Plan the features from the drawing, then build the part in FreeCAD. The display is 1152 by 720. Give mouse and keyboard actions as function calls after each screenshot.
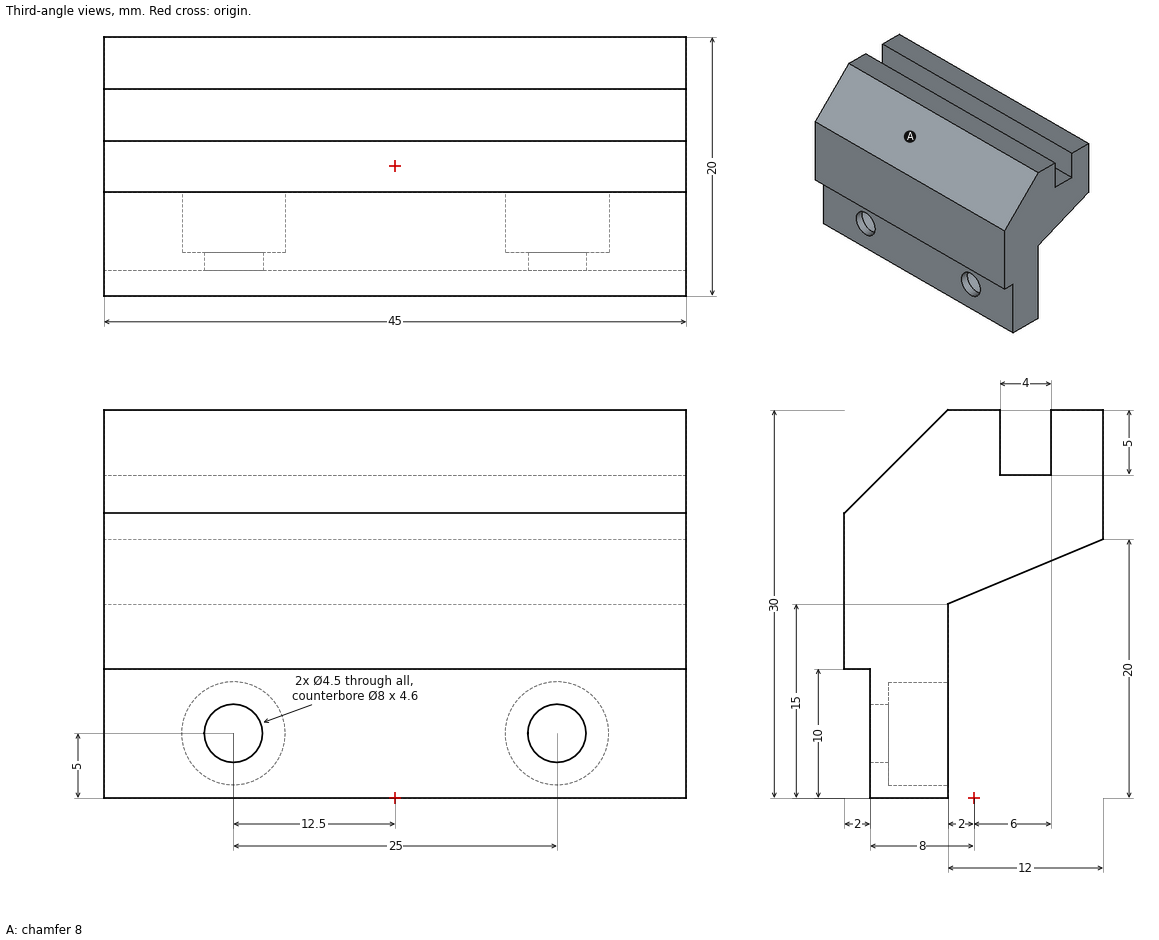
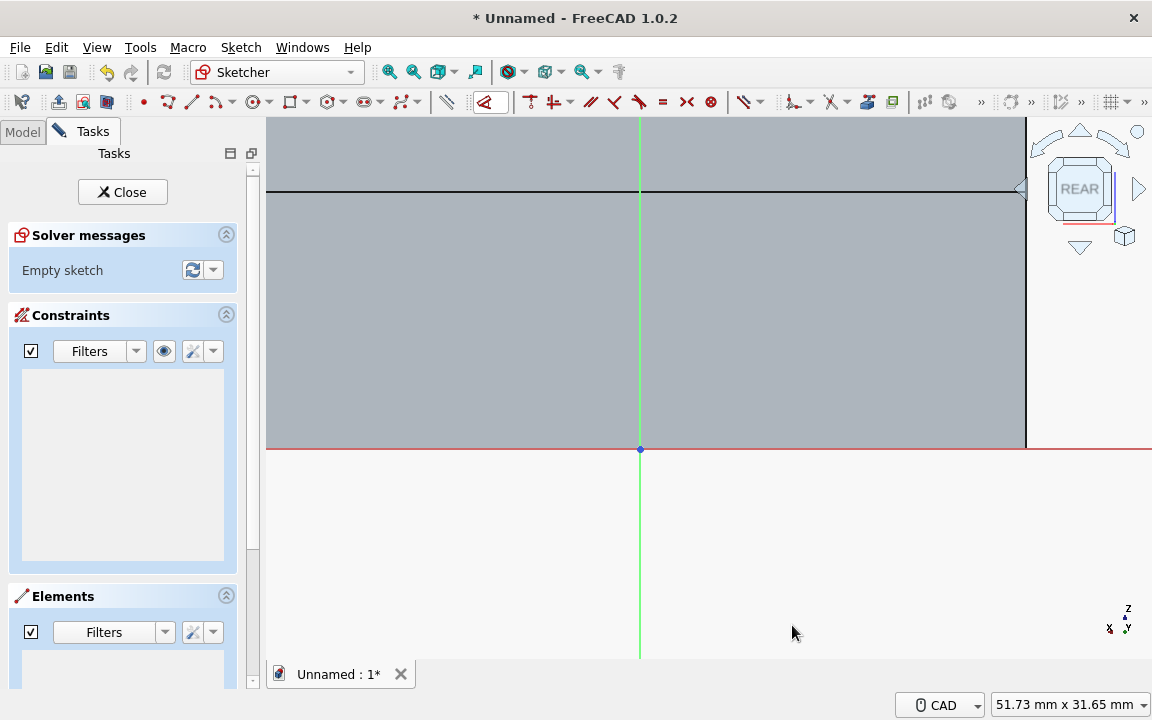
click(254, 102)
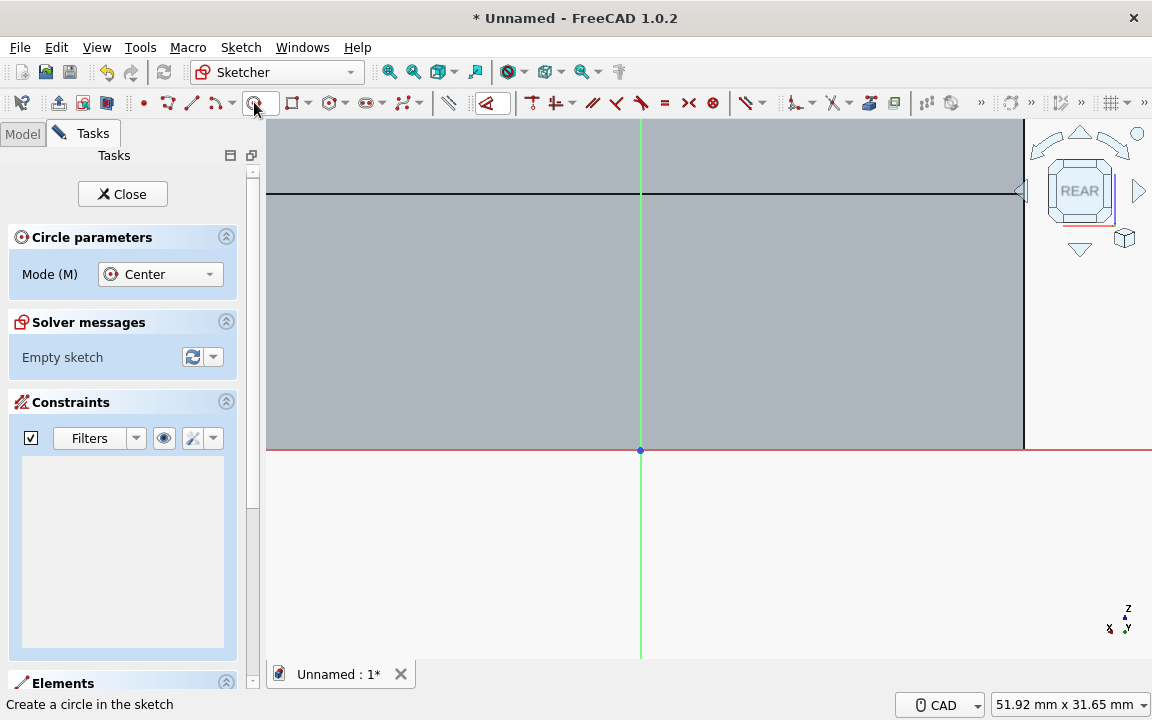
click(854, 365)
move(881, 338)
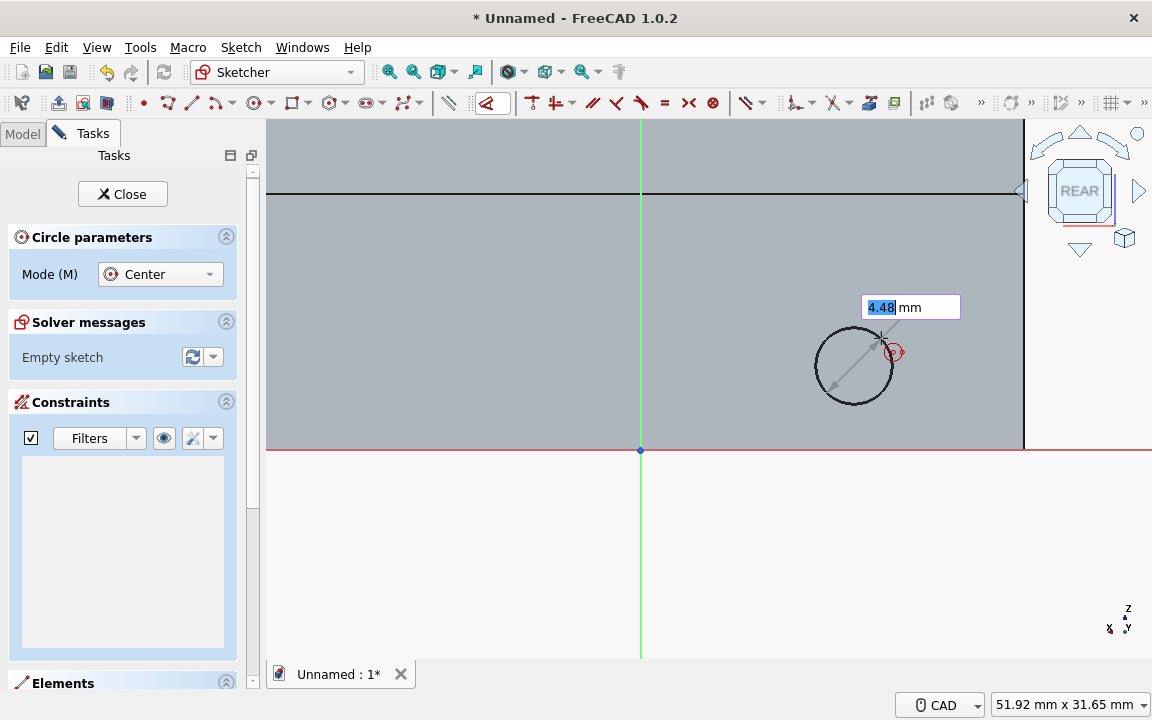
text(4.5)
key(Return)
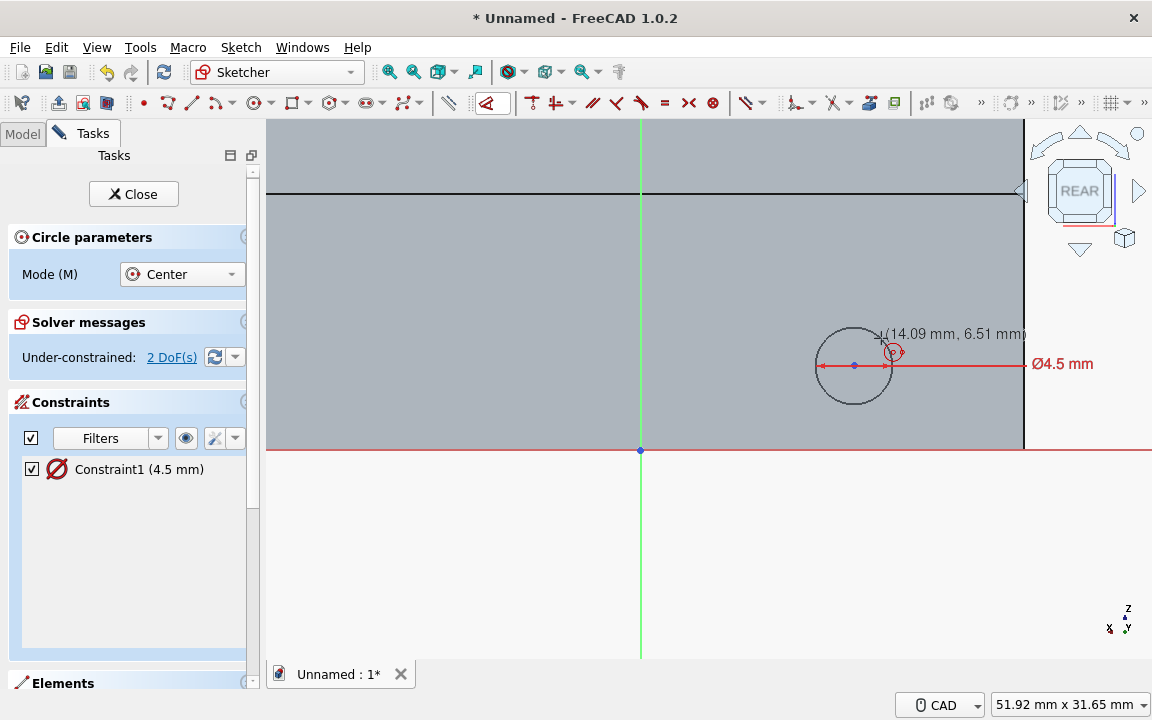
click(427, 365)
move(454, 338)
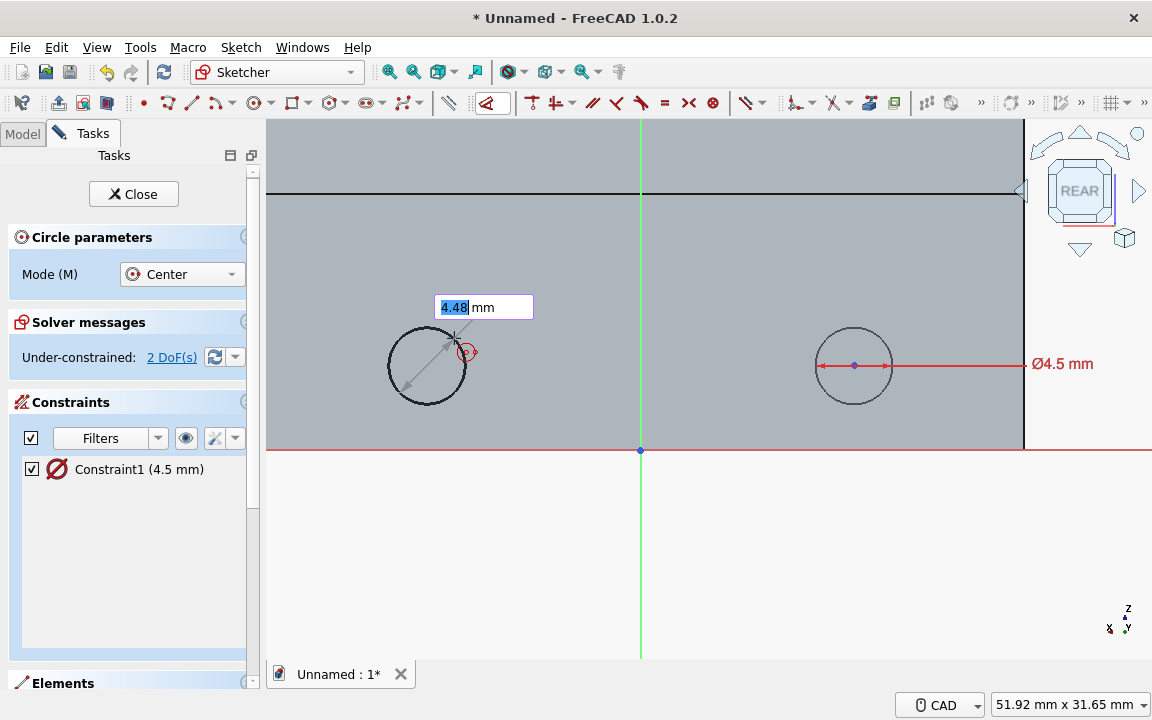
text(4.5)
key(Return)
key(Escape)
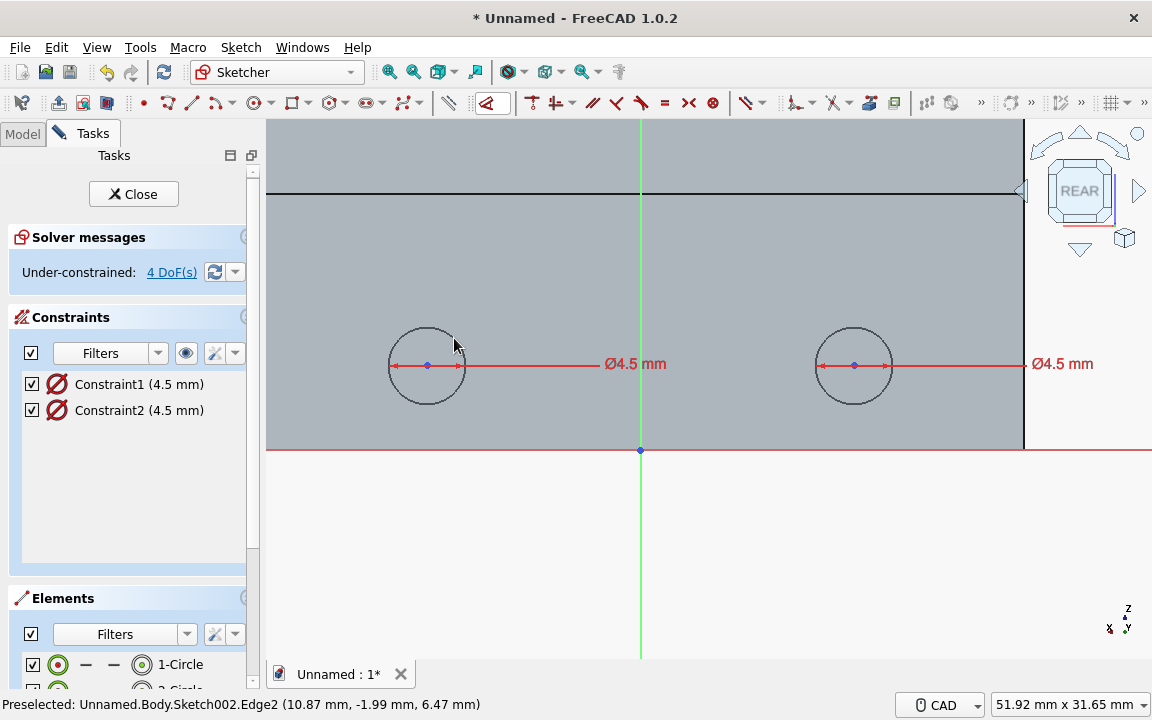
click(854, 366)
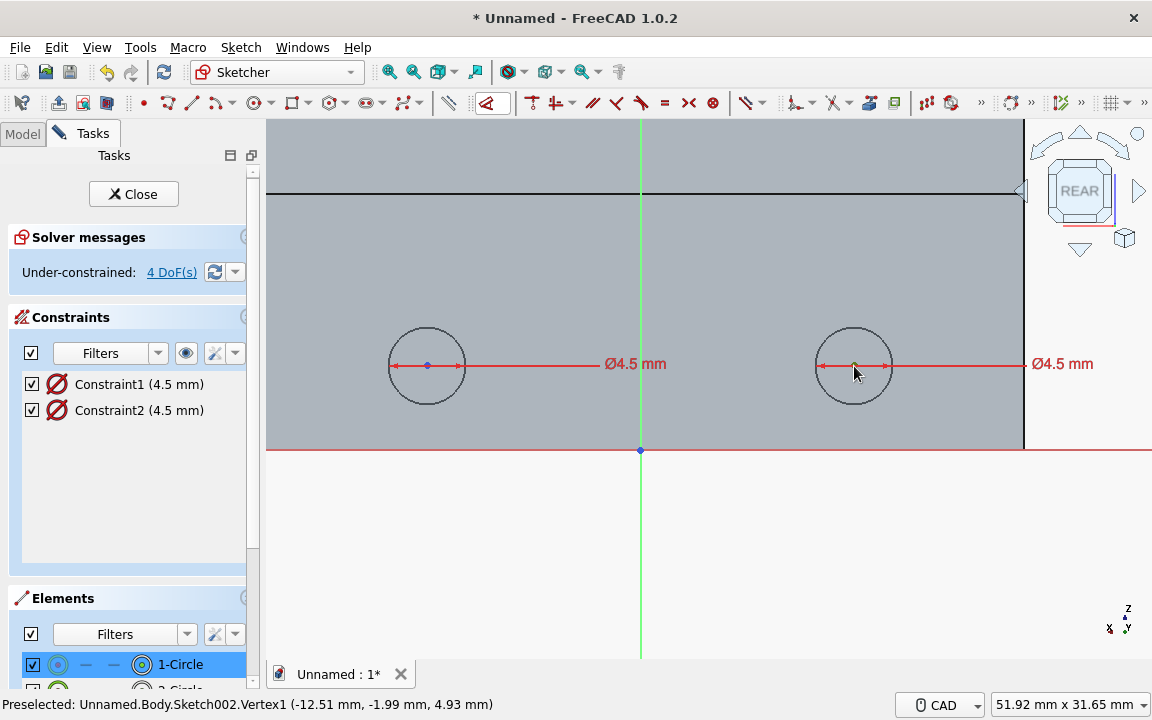
click(427, 366)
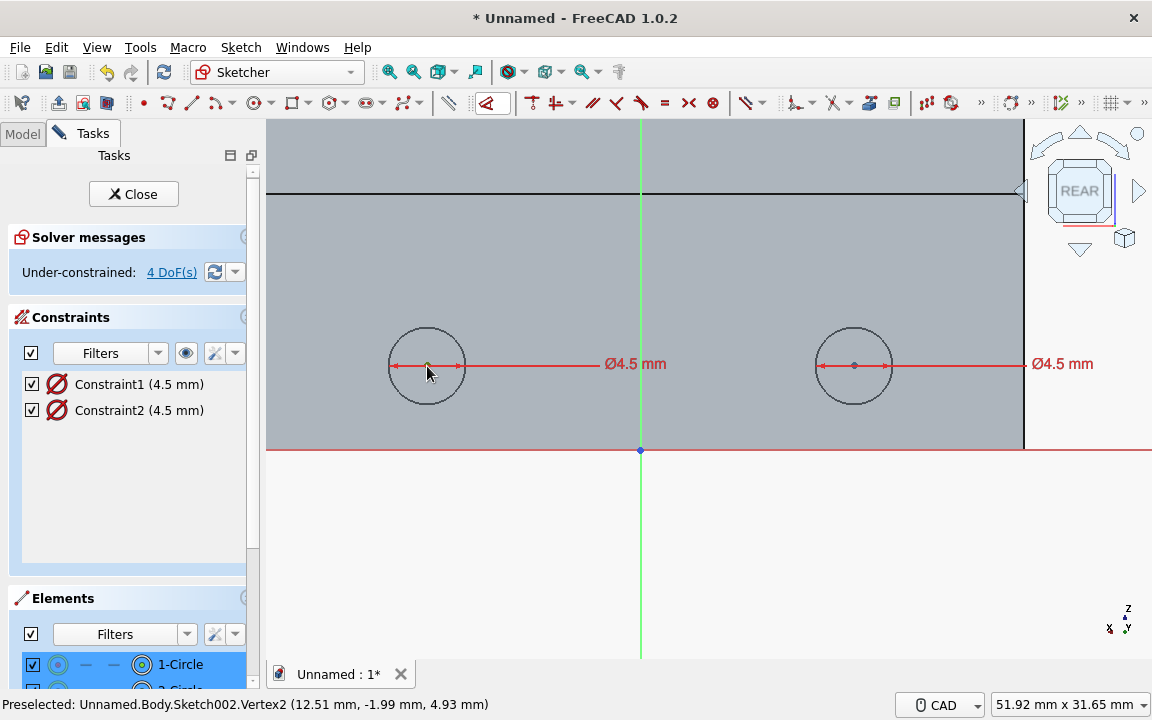
key(h)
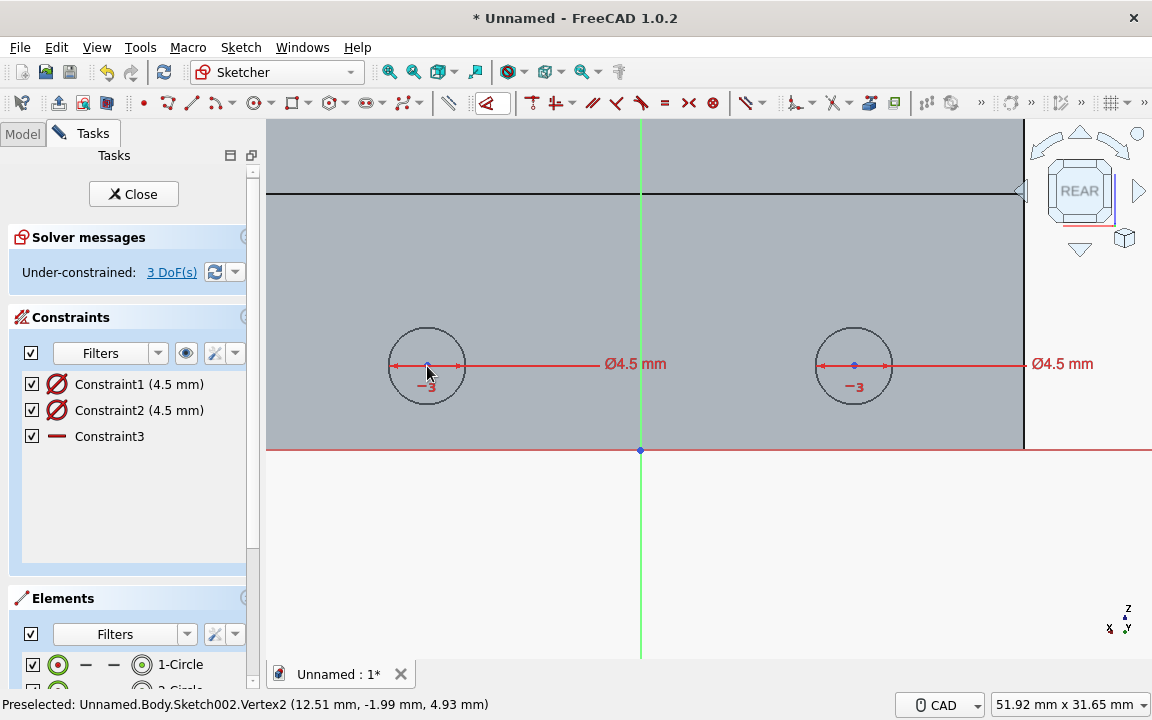
click(854, 366)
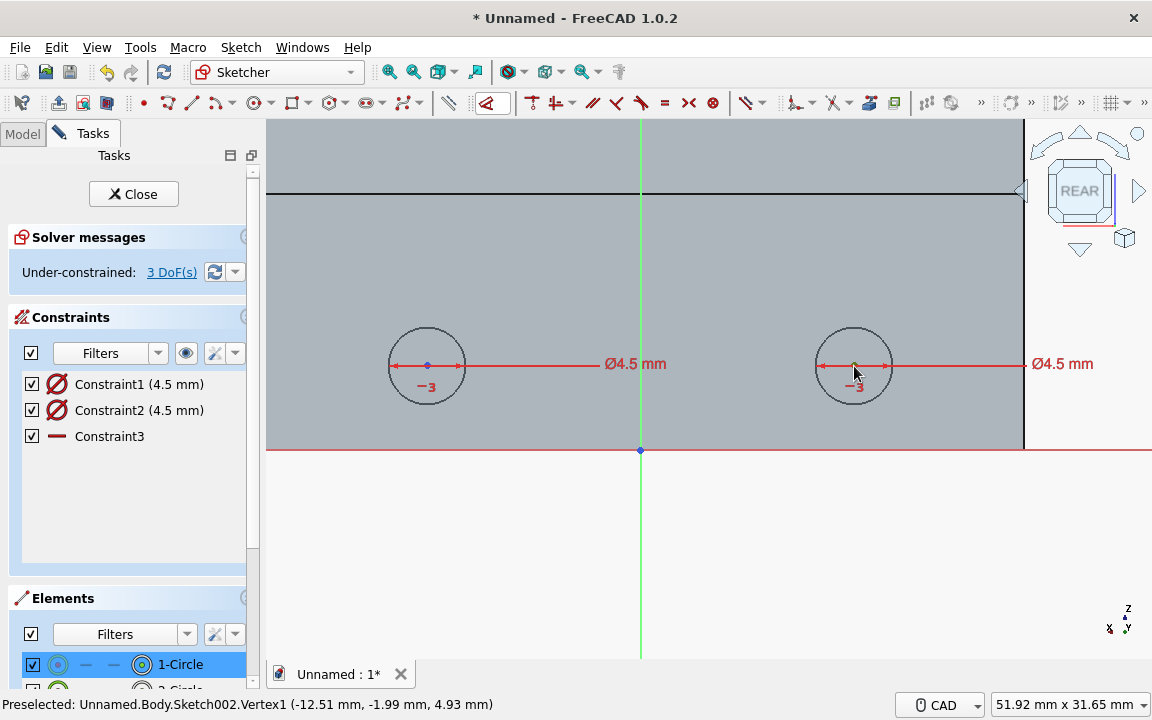
key(i)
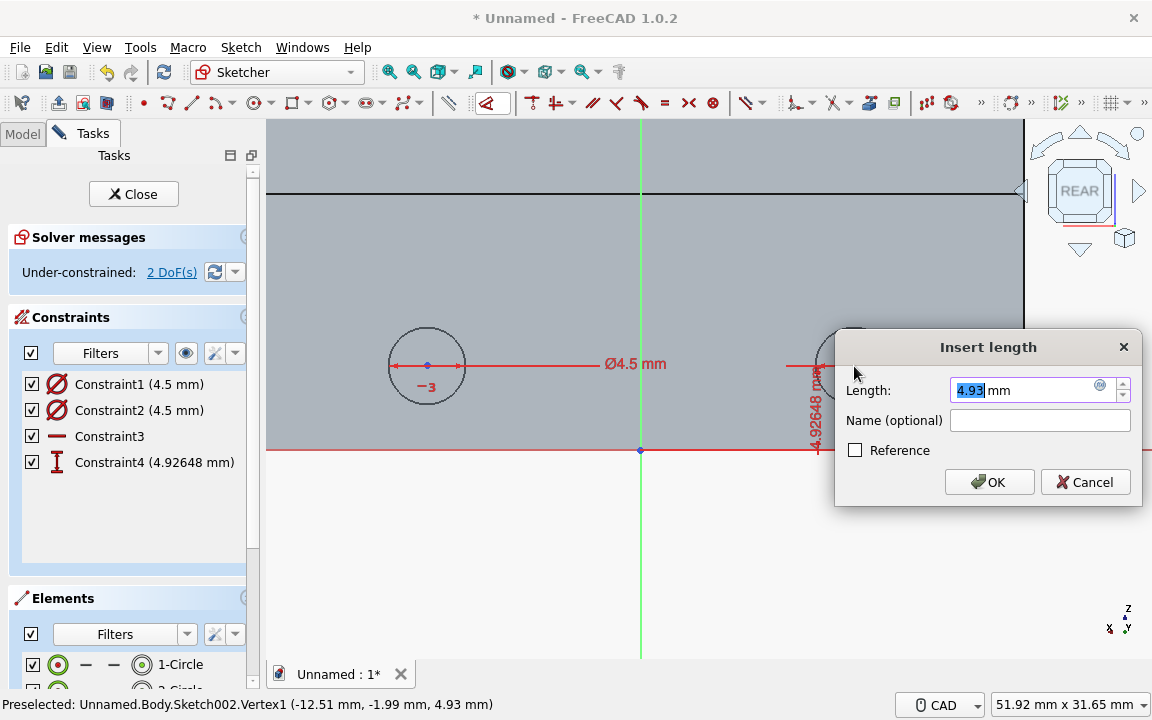
text(5)
key(Return)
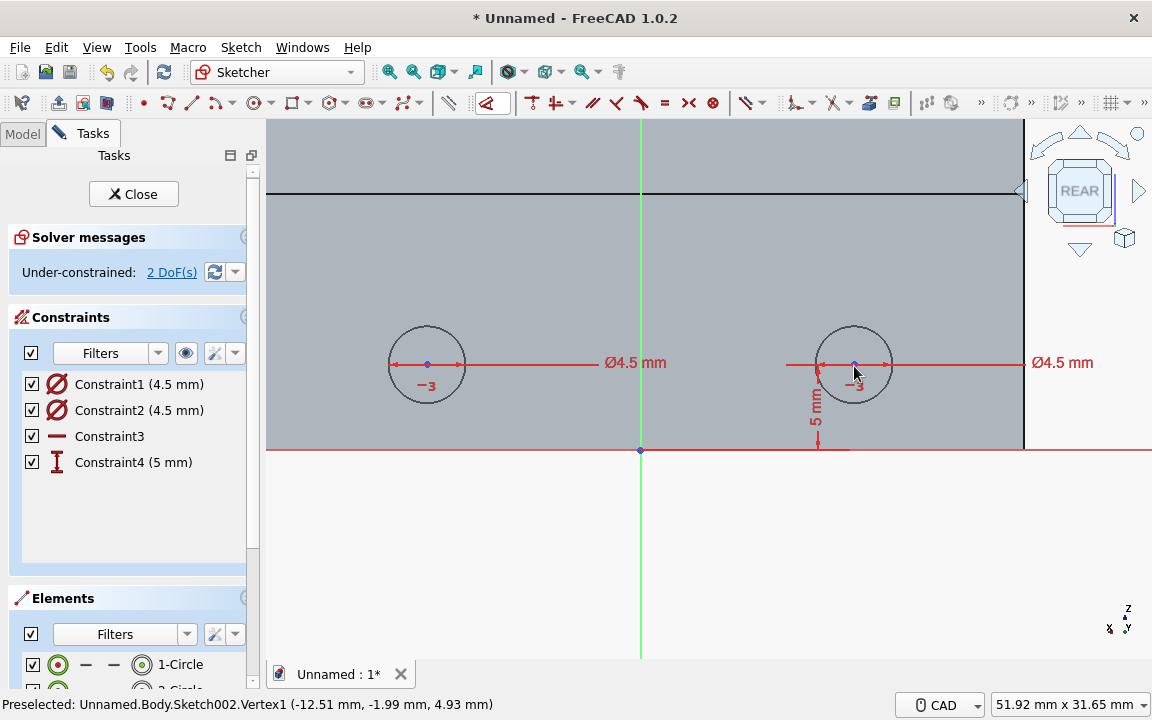
click(854, 365)